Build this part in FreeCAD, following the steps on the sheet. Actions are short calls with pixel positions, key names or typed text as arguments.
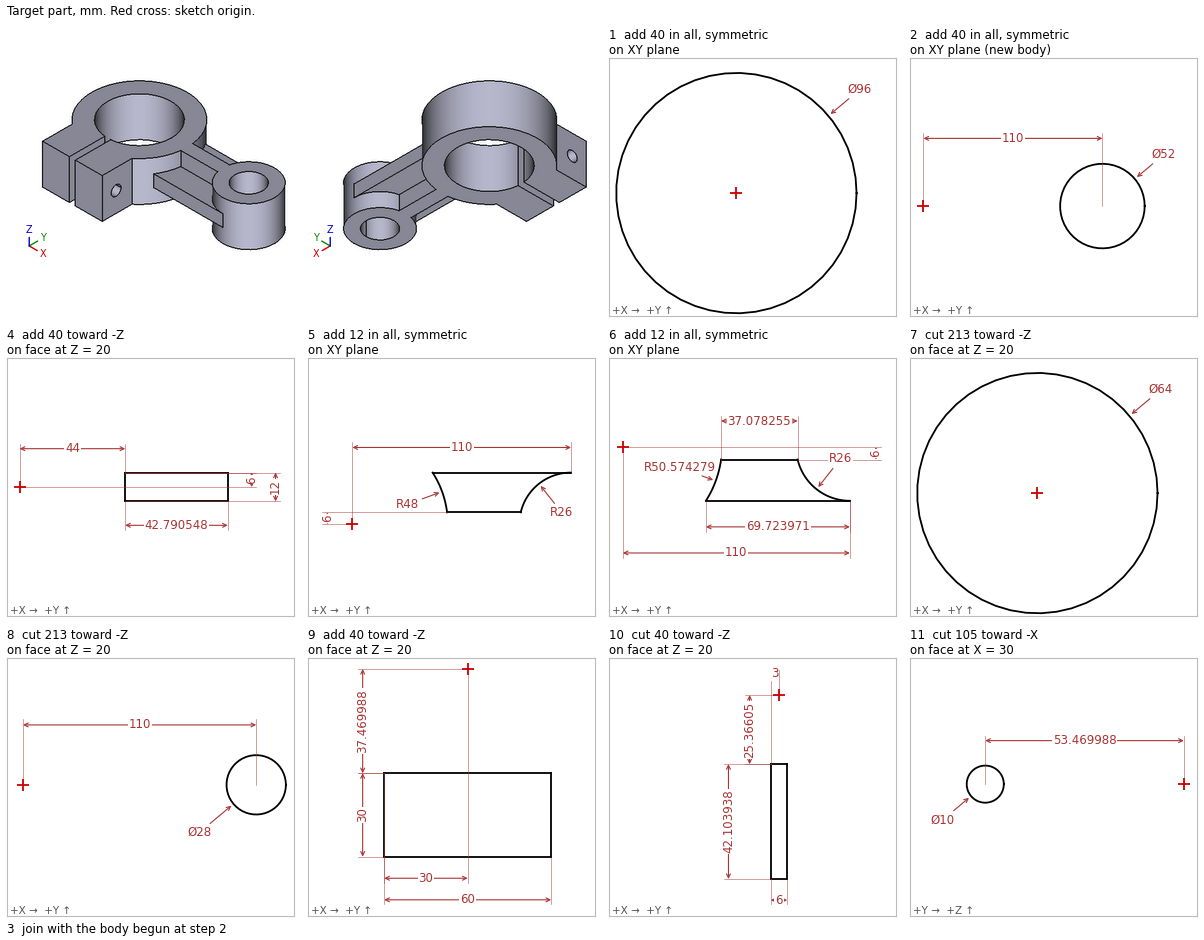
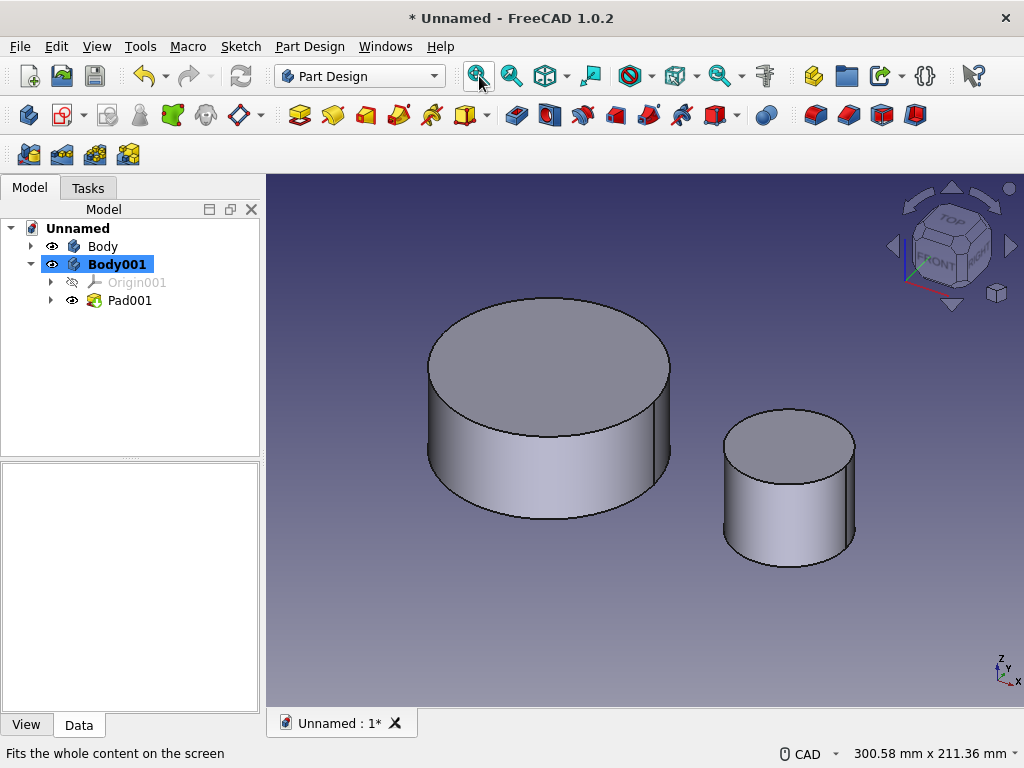
double_click(97, 246)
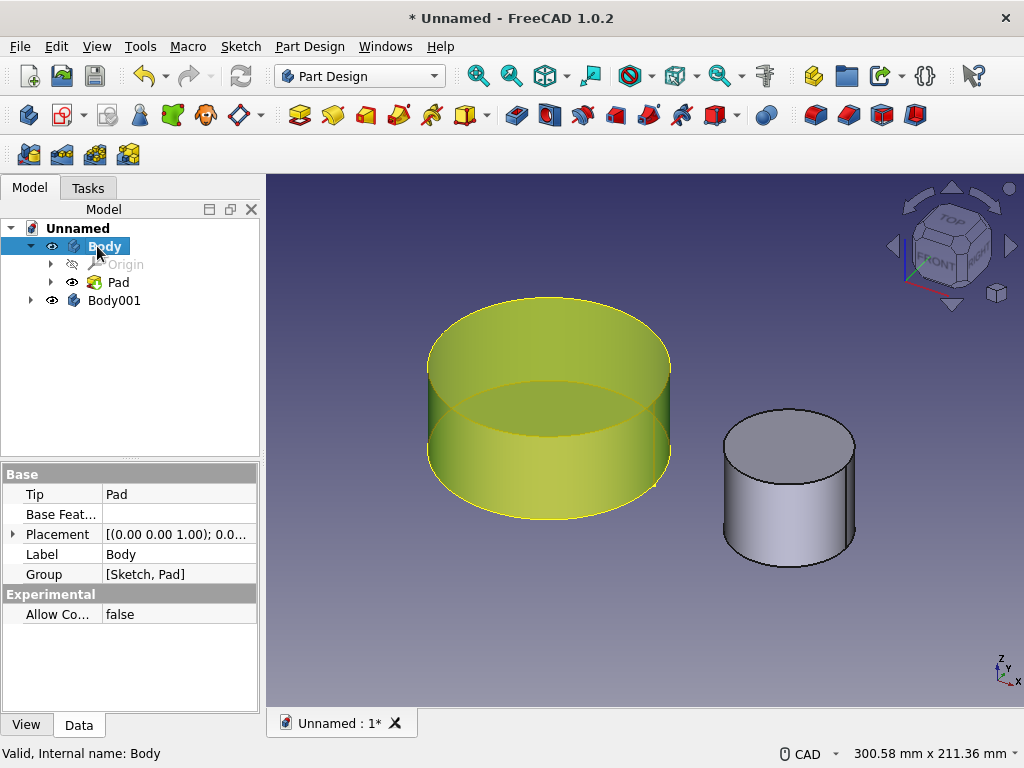
click(97, 246)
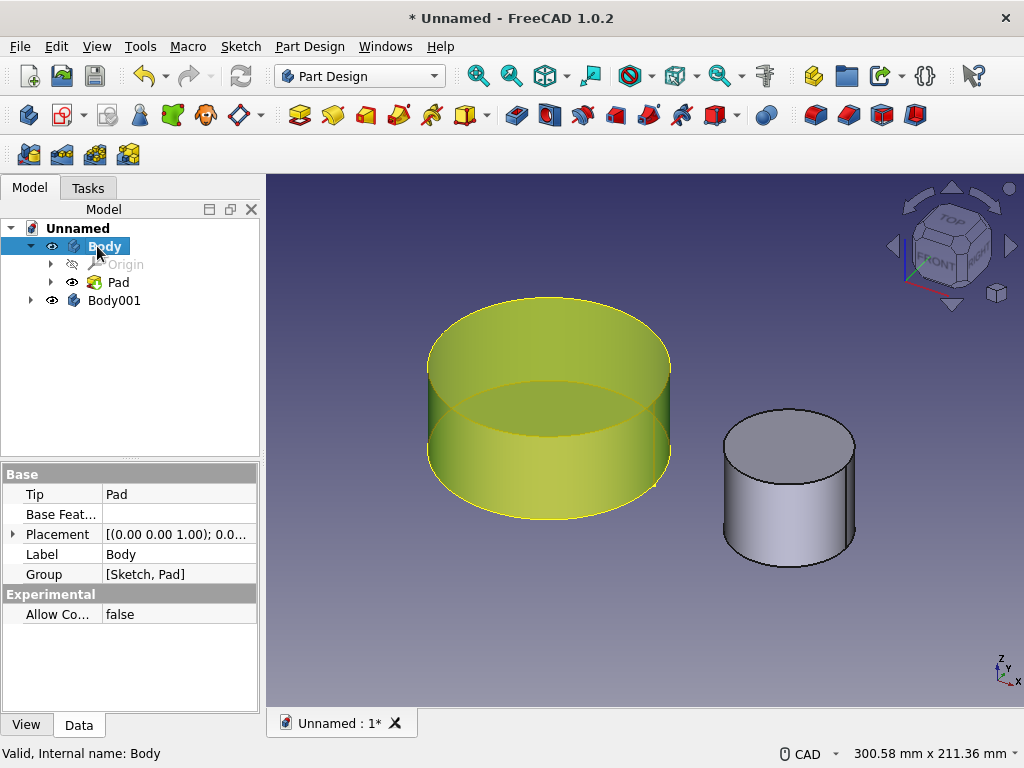
click(148, 614)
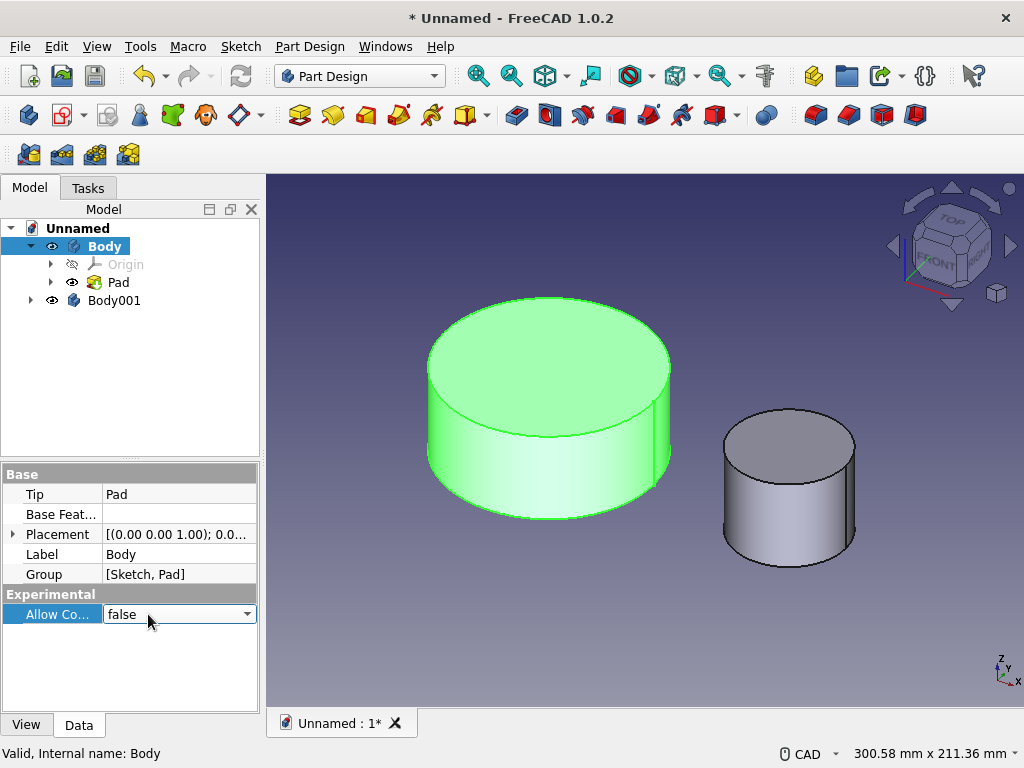
click(148, 614)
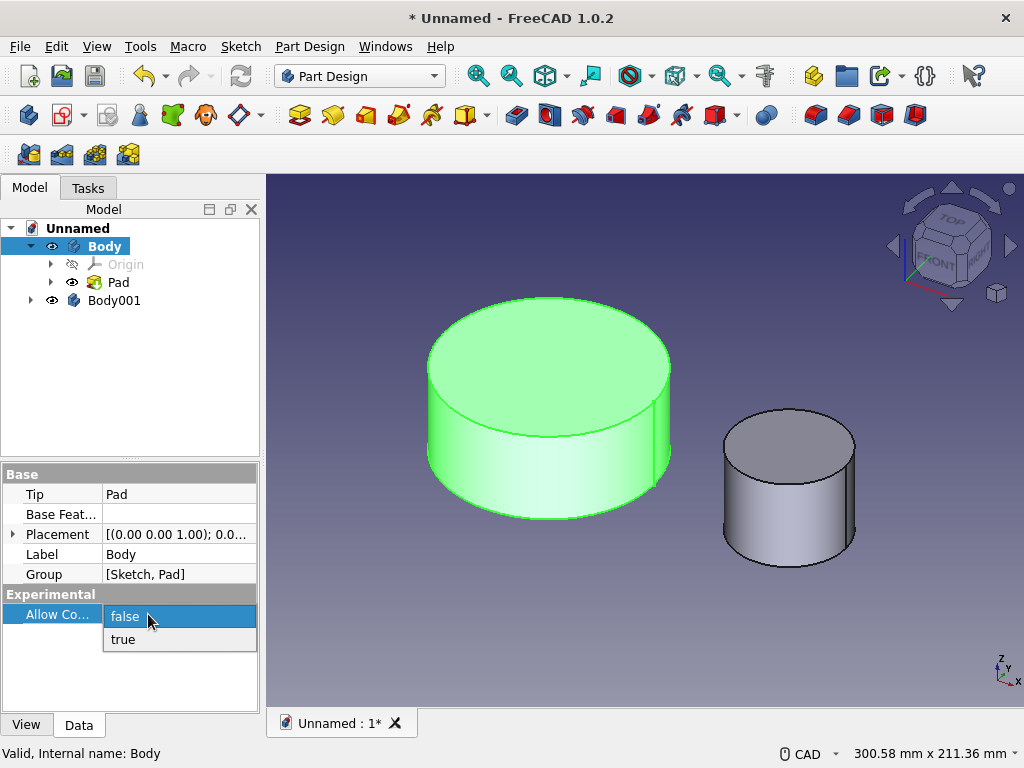
click(178, 640)
key(Return)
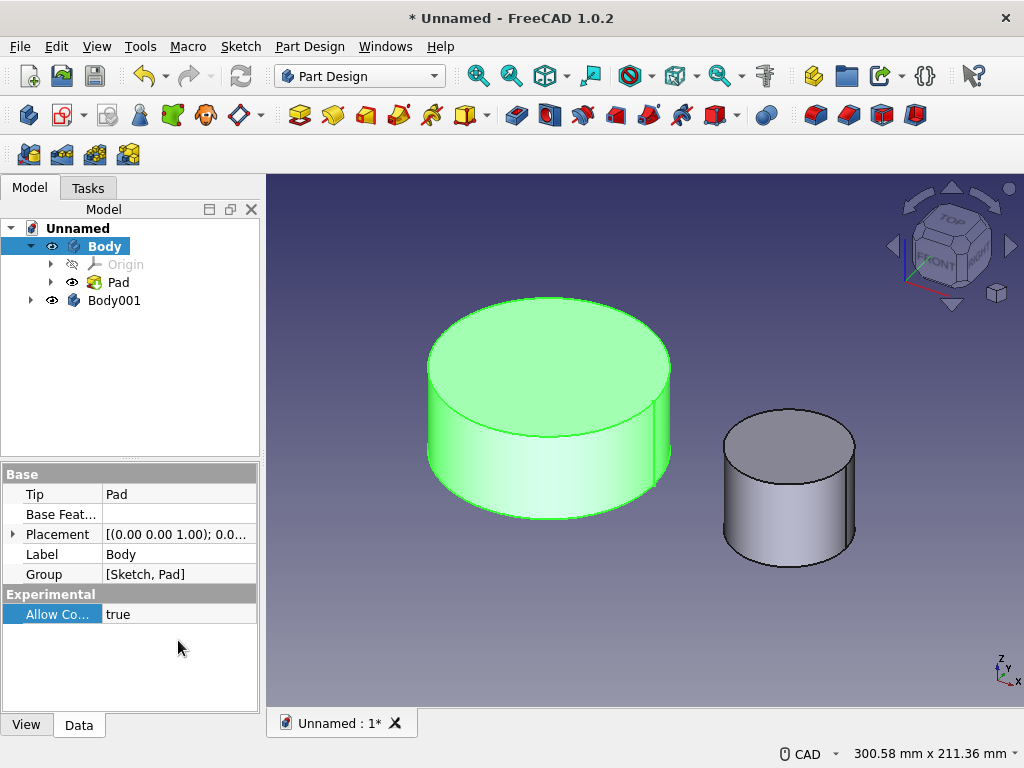
click(97, 300)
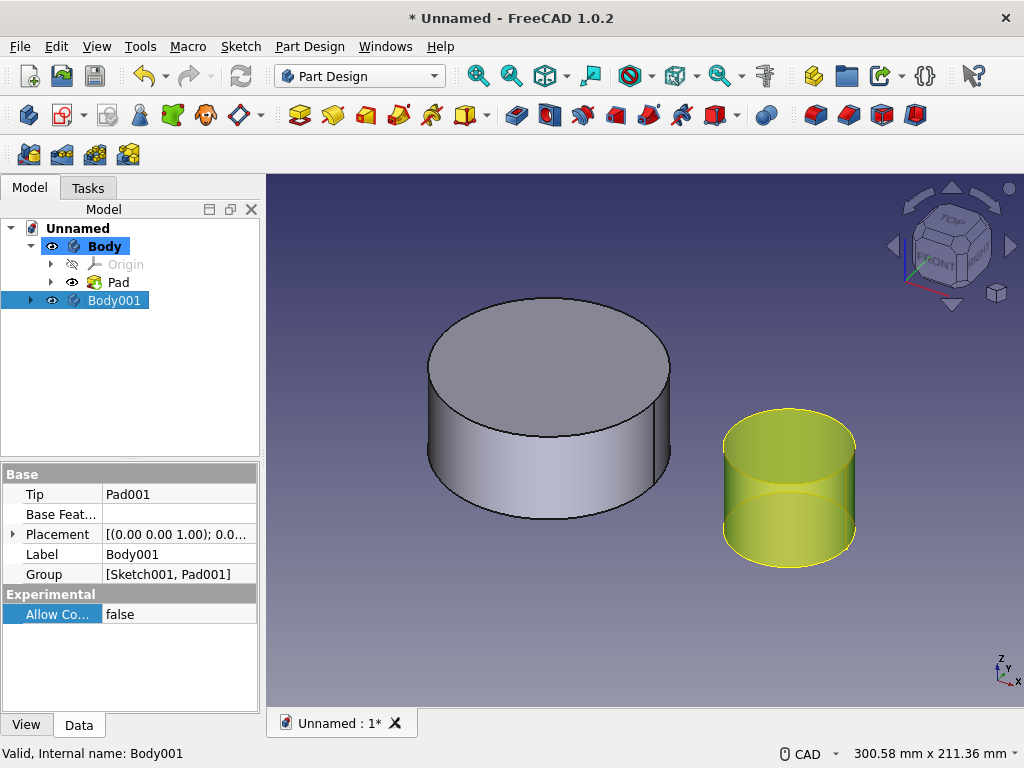
click(767, 116)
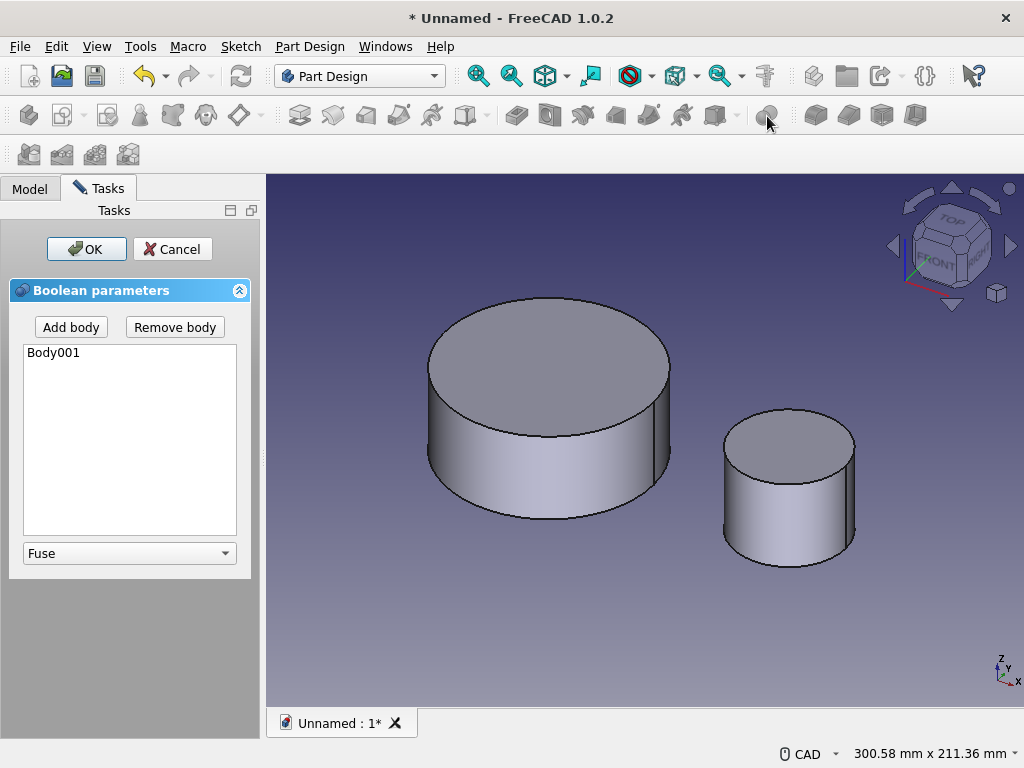
click(87, 249)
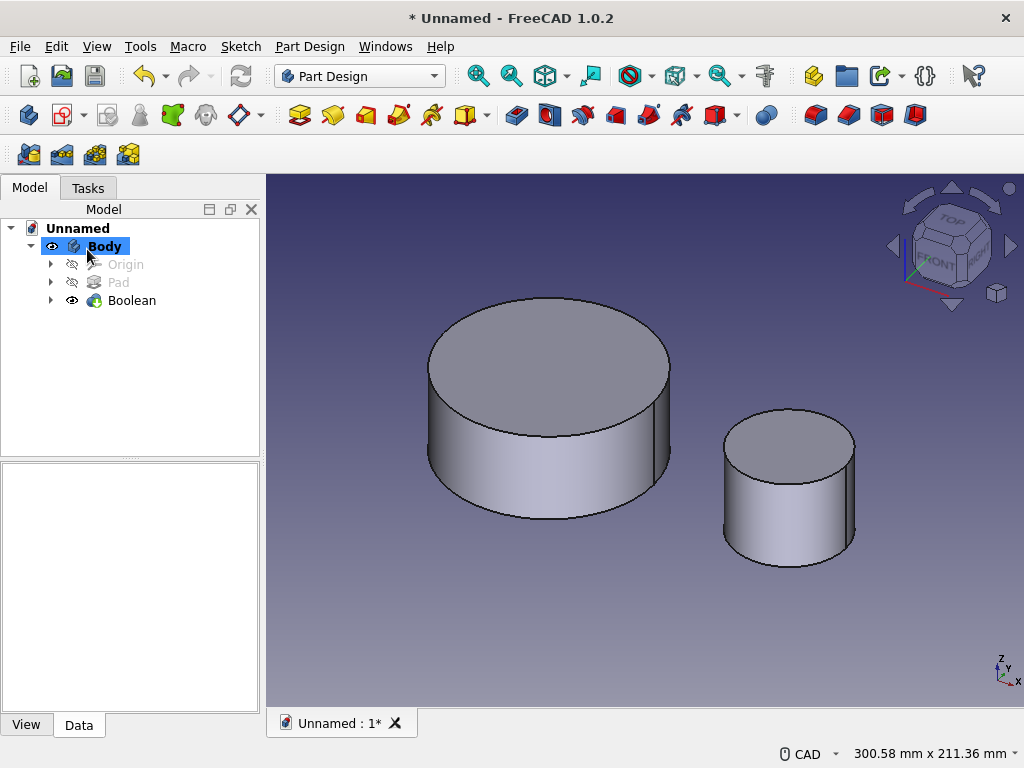
click(549, 366)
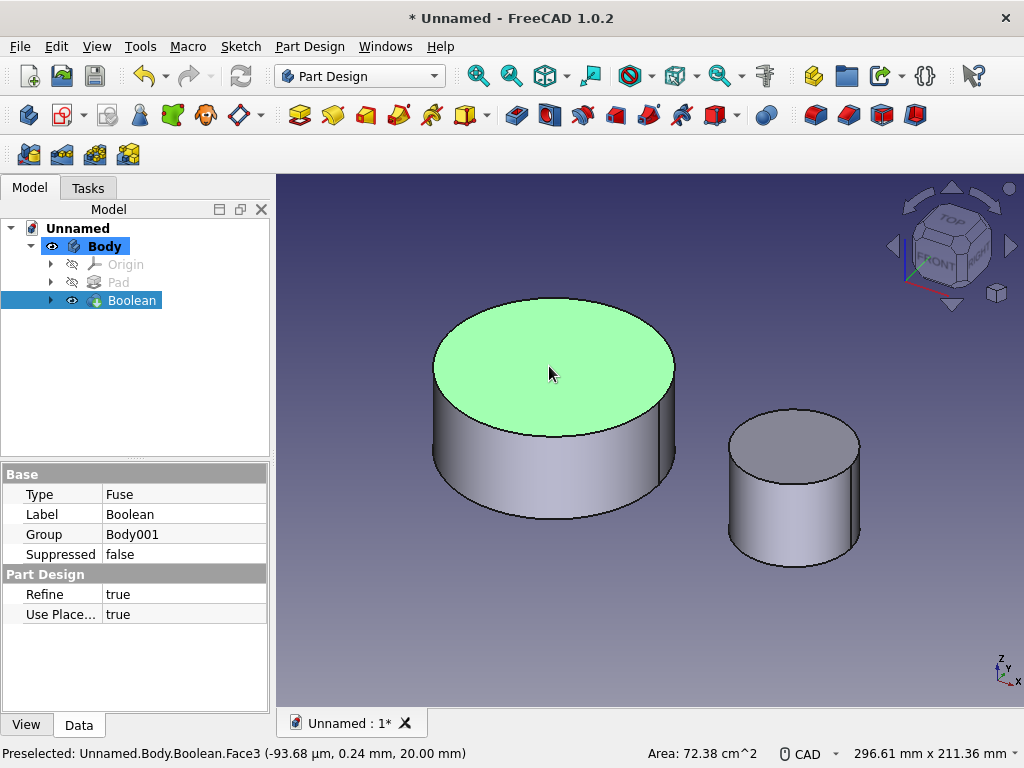
click(62, 116)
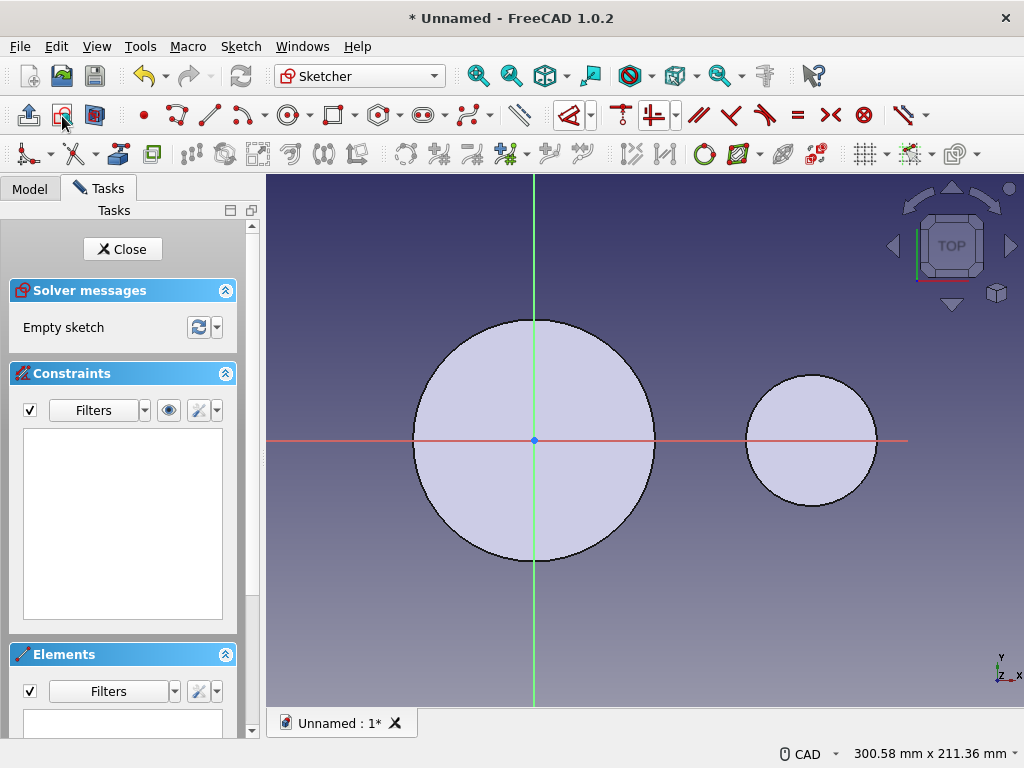
scroll(725, 441, up, 3)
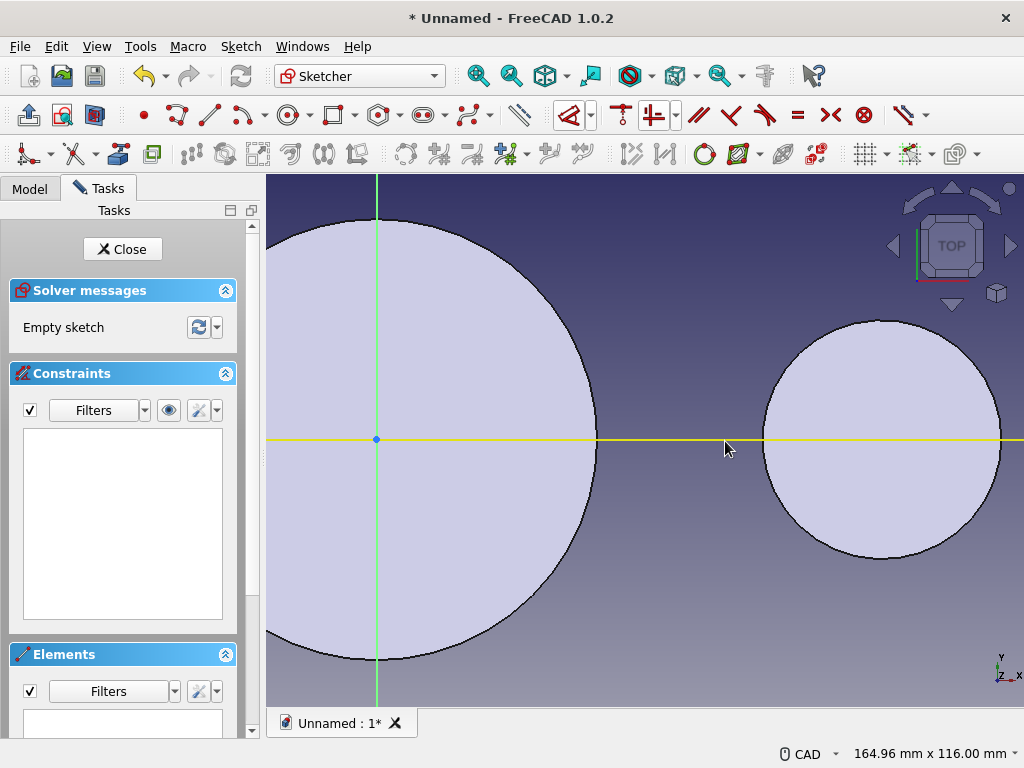
click(332, 116)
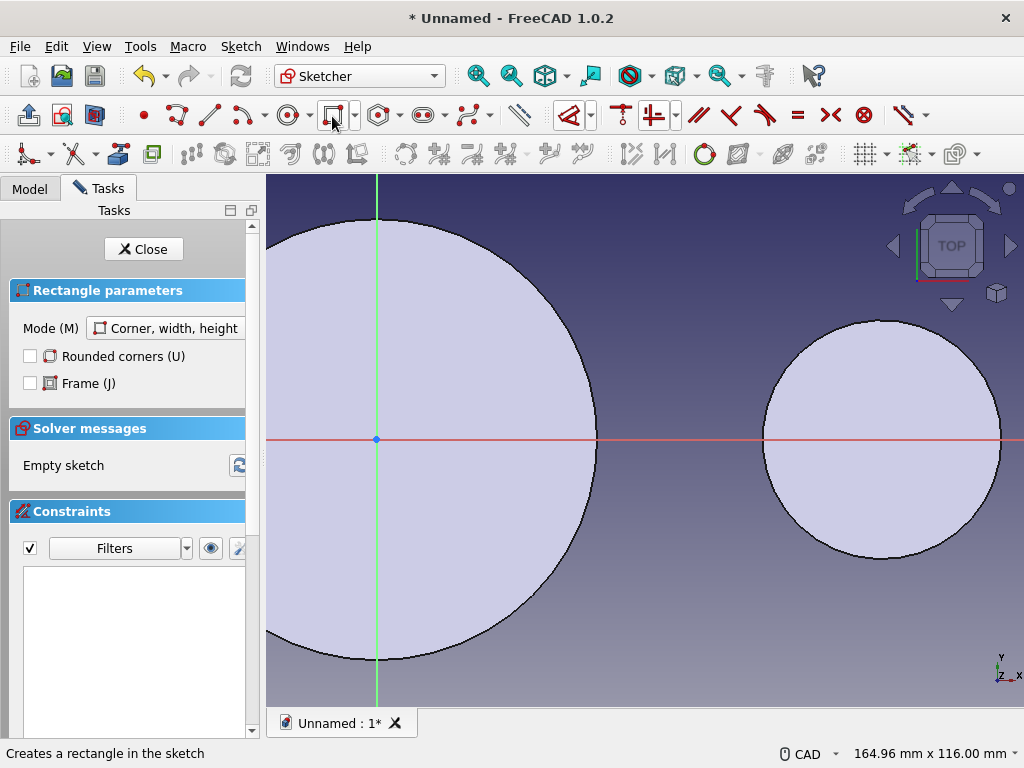
click(579, 412)
click(775, 467)
key(Escape)